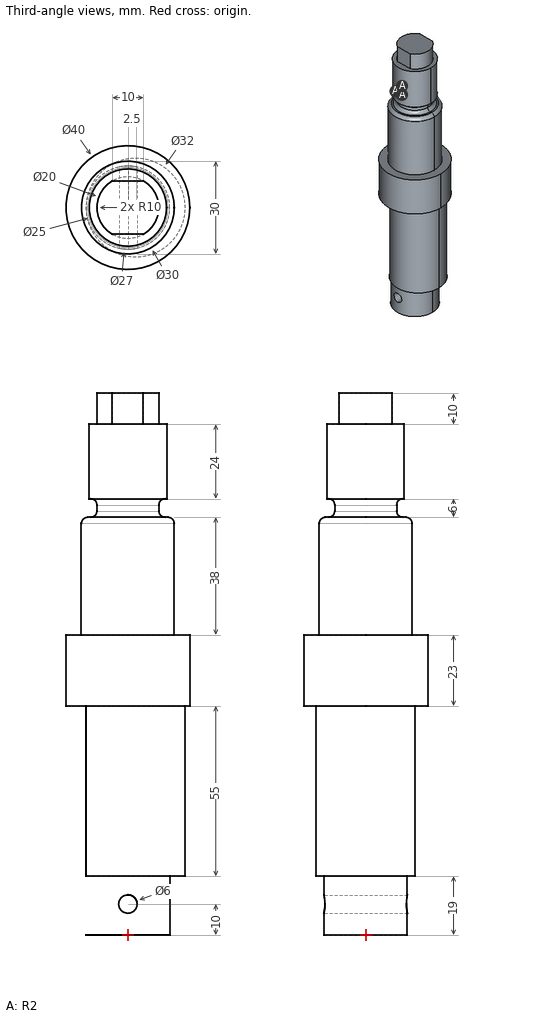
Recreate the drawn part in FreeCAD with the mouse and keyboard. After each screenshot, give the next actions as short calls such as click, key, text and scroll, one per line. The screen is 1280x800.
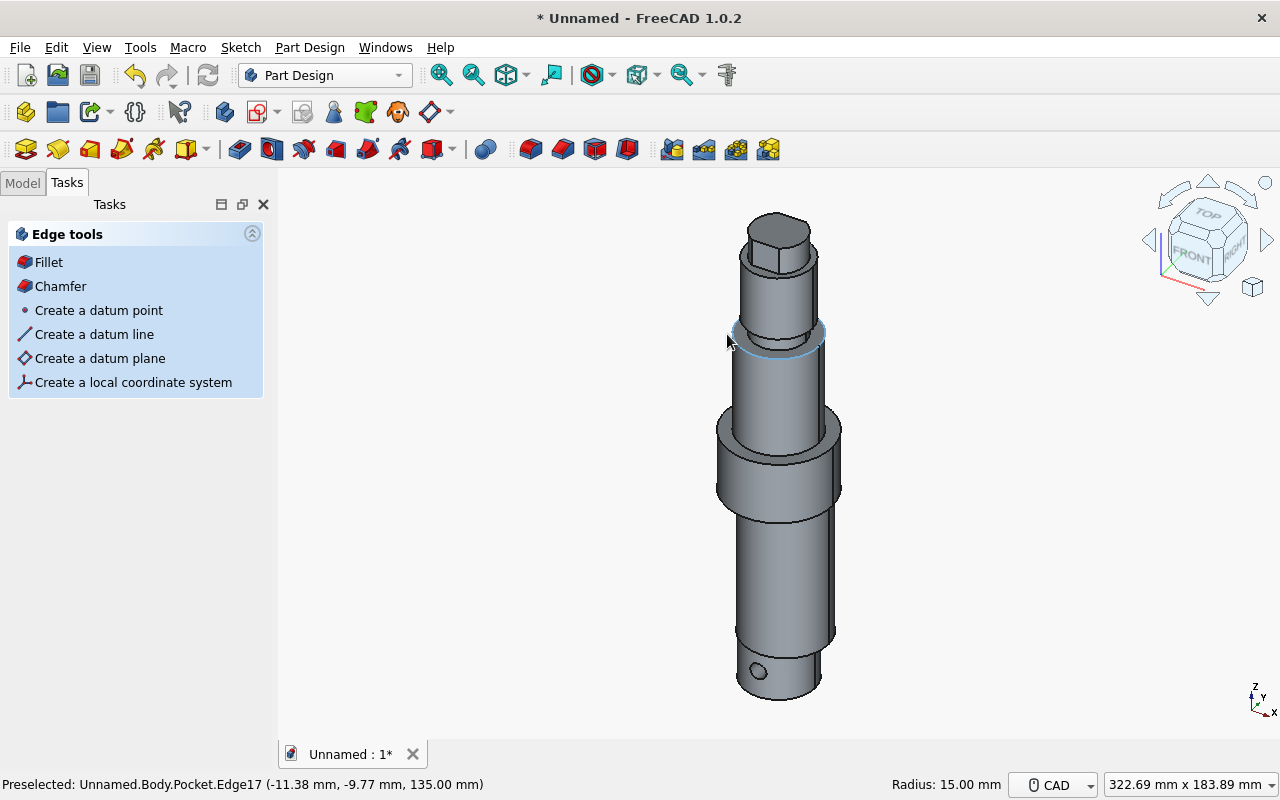
key(0)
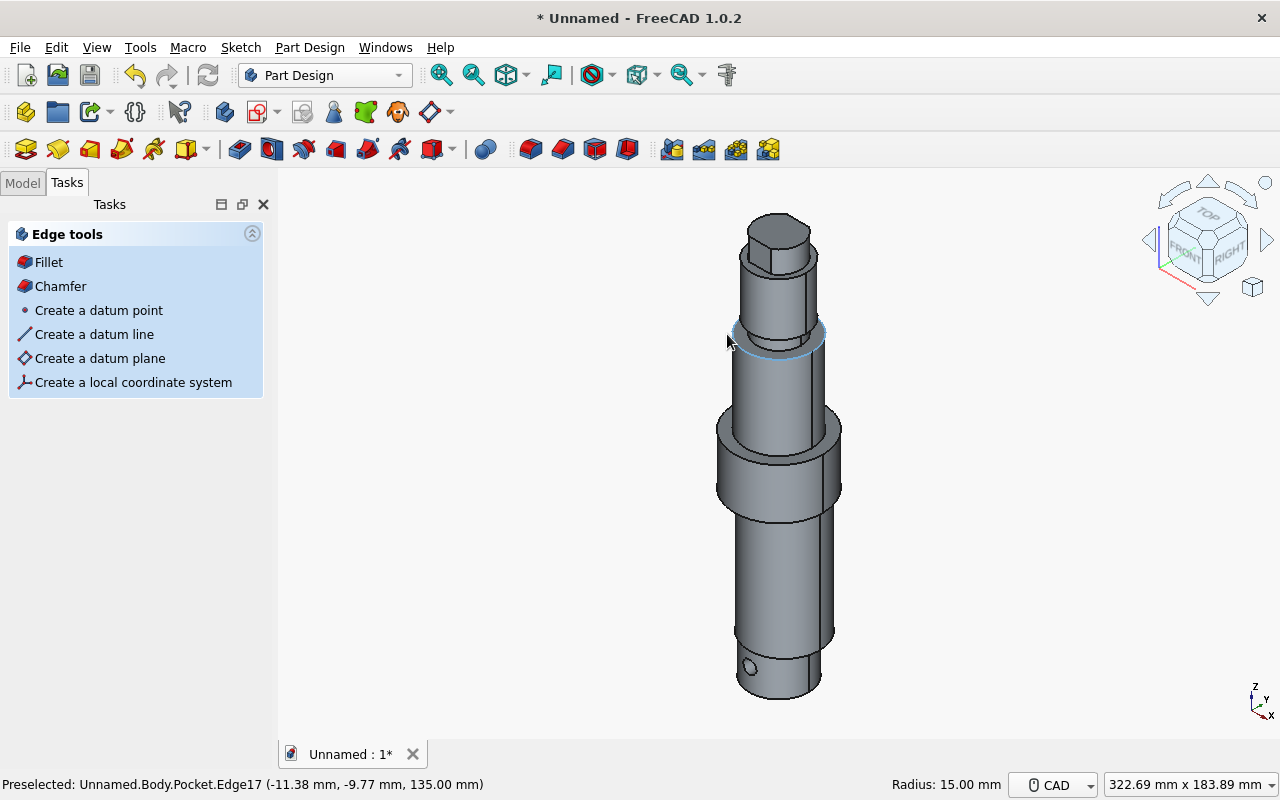
key(2)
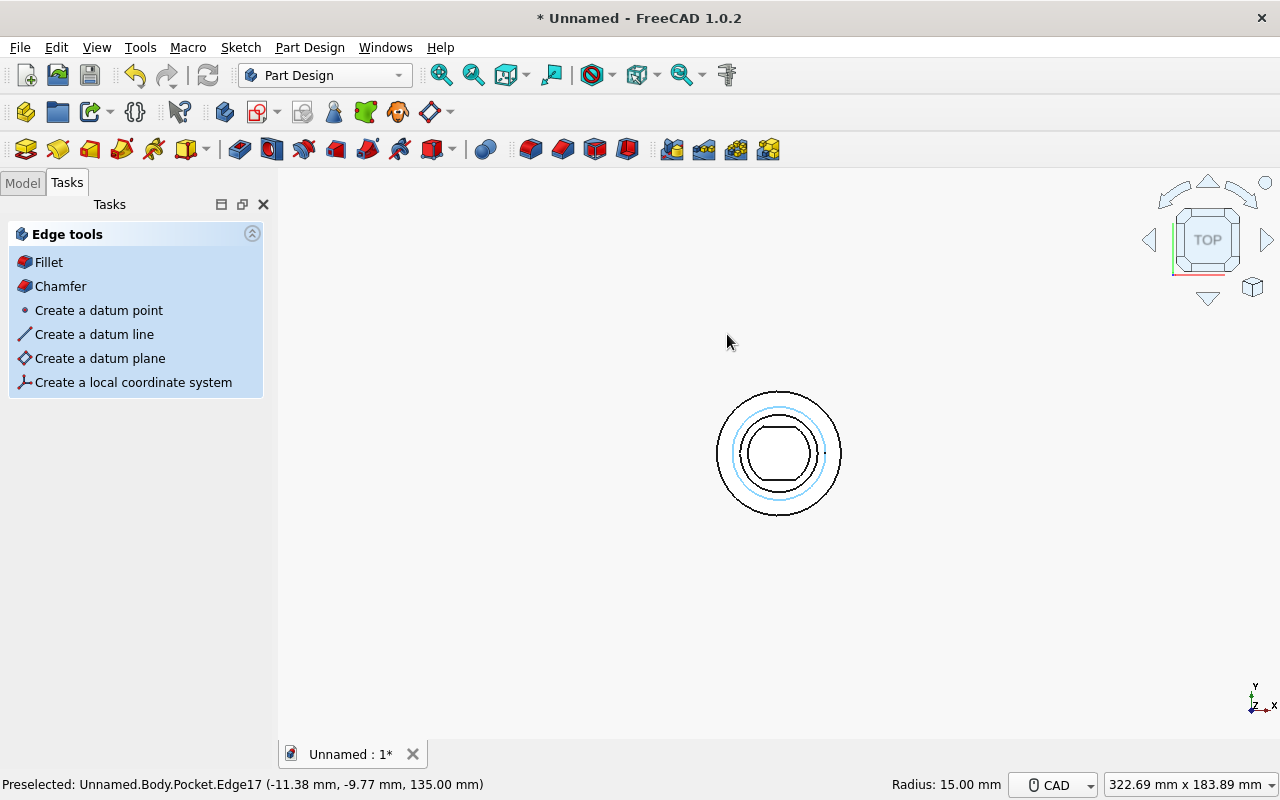
key(v)
key(f)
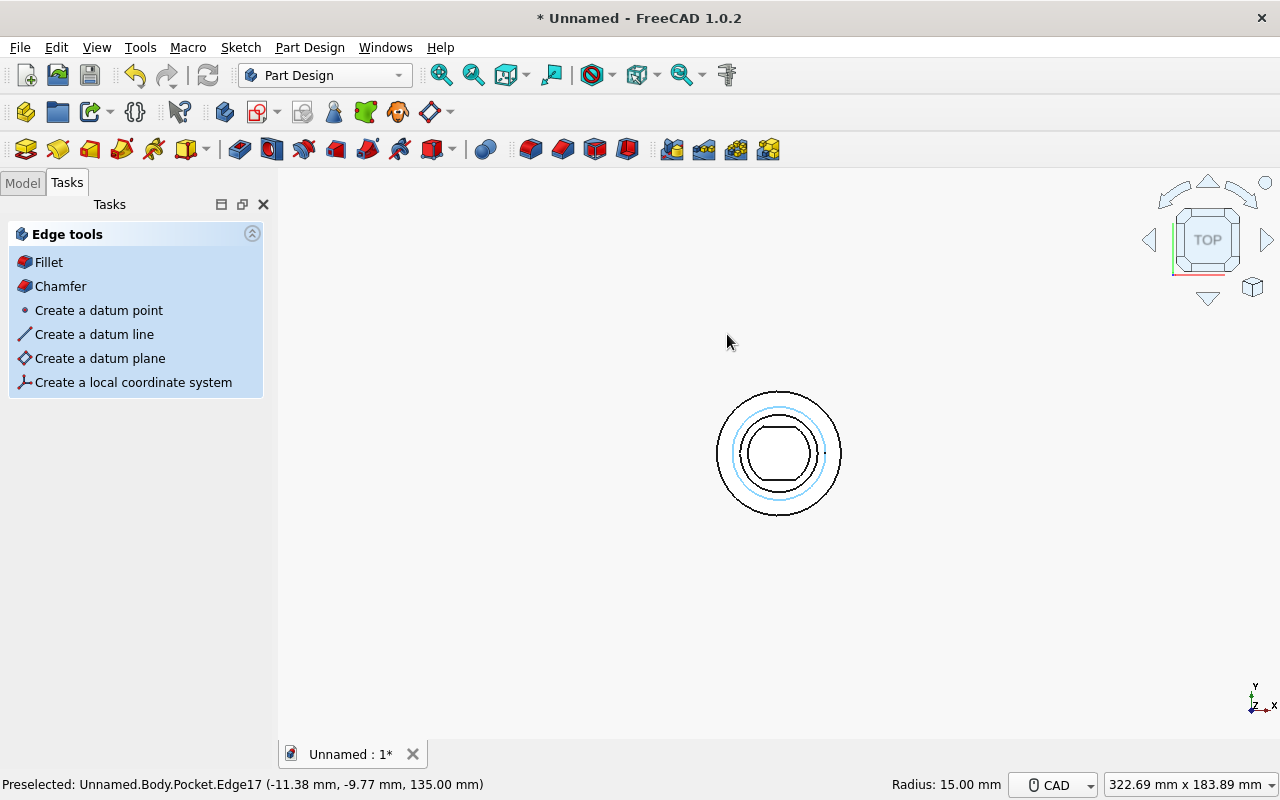
key(1)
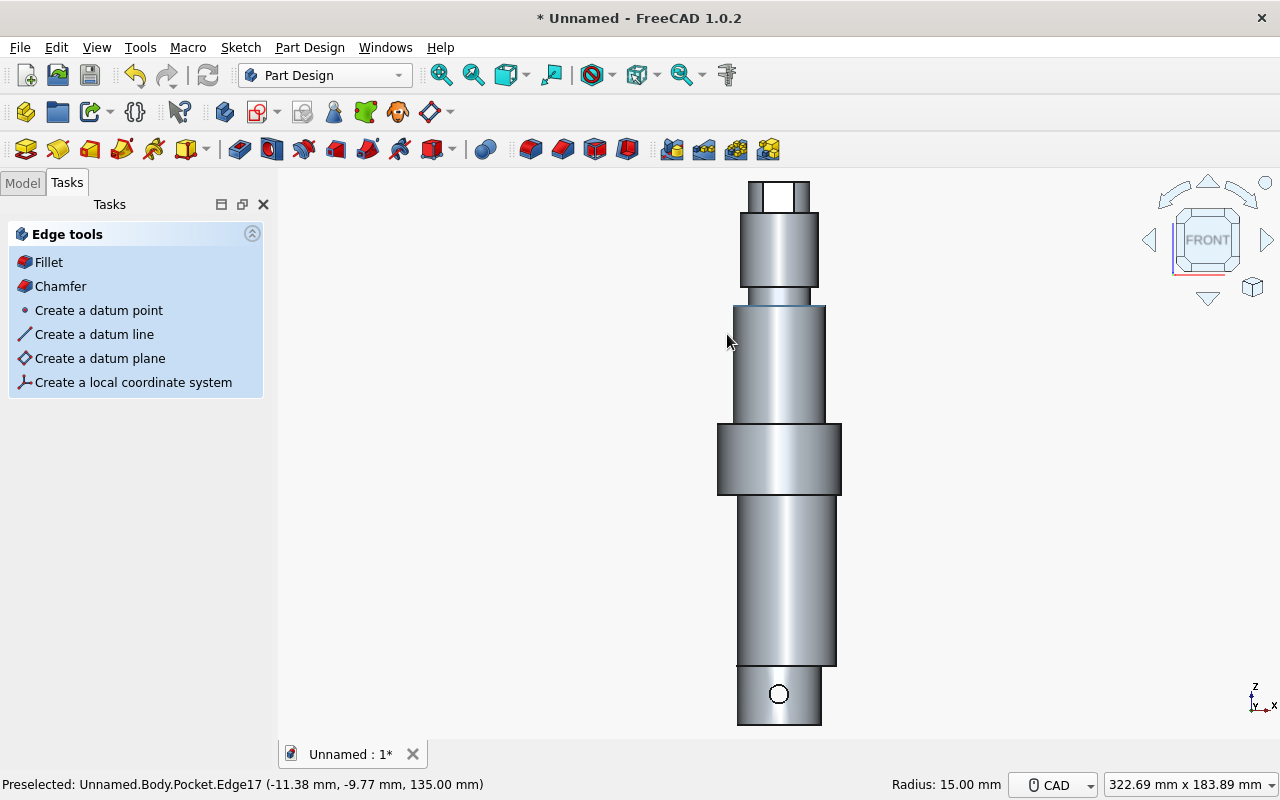
key(3)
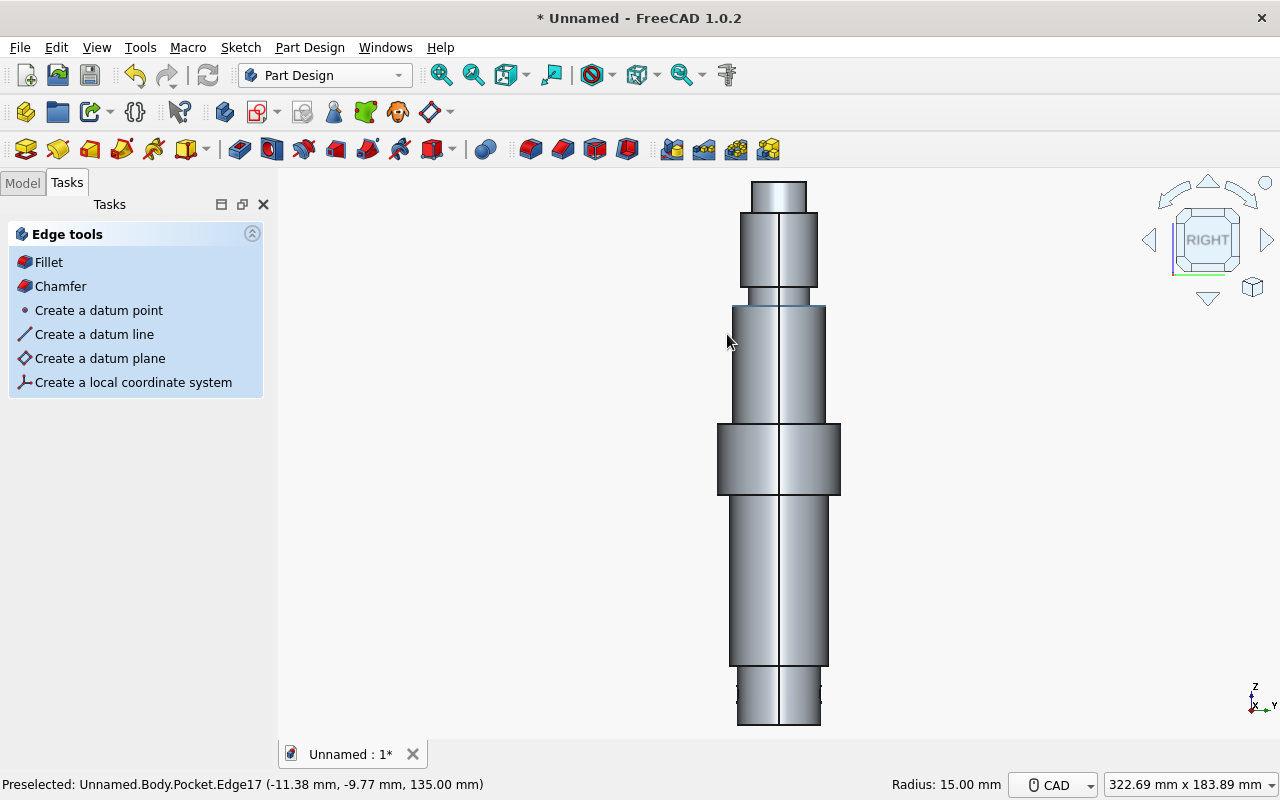
key(5)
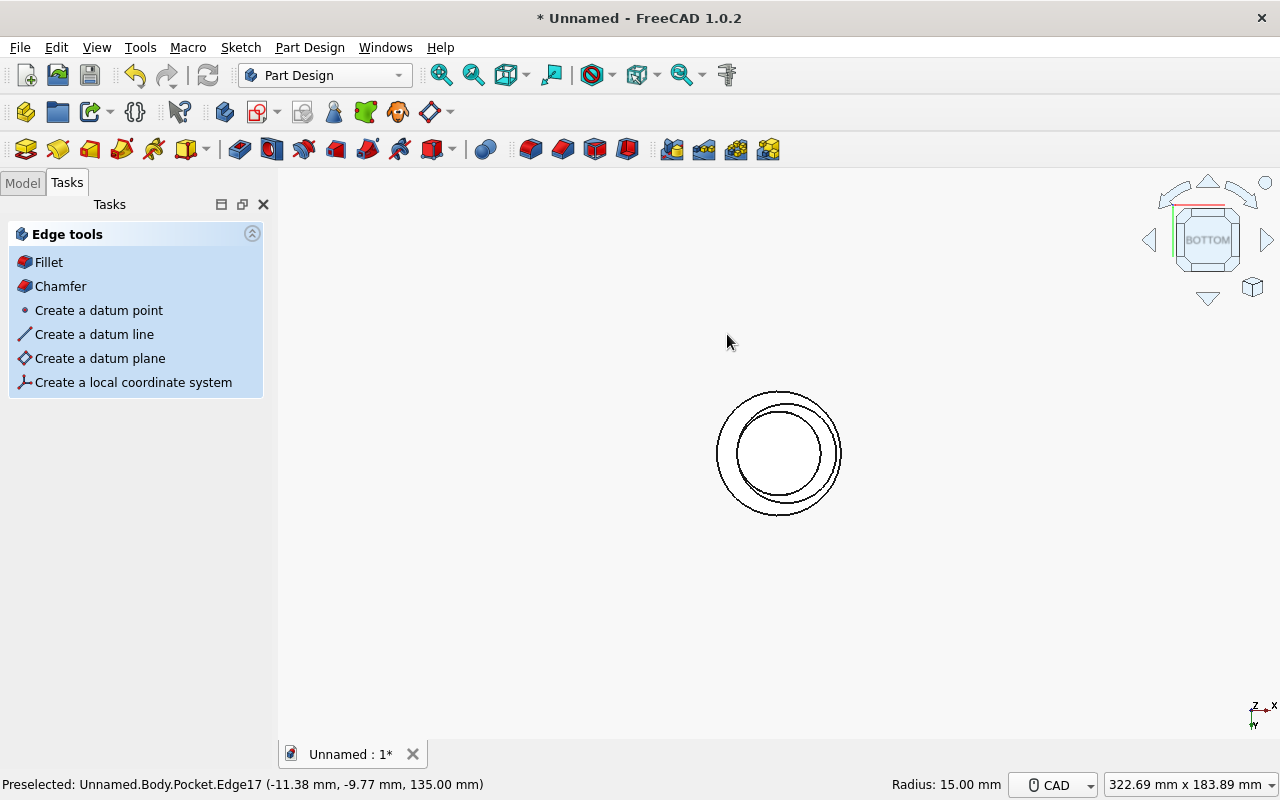
key(v)
key(f)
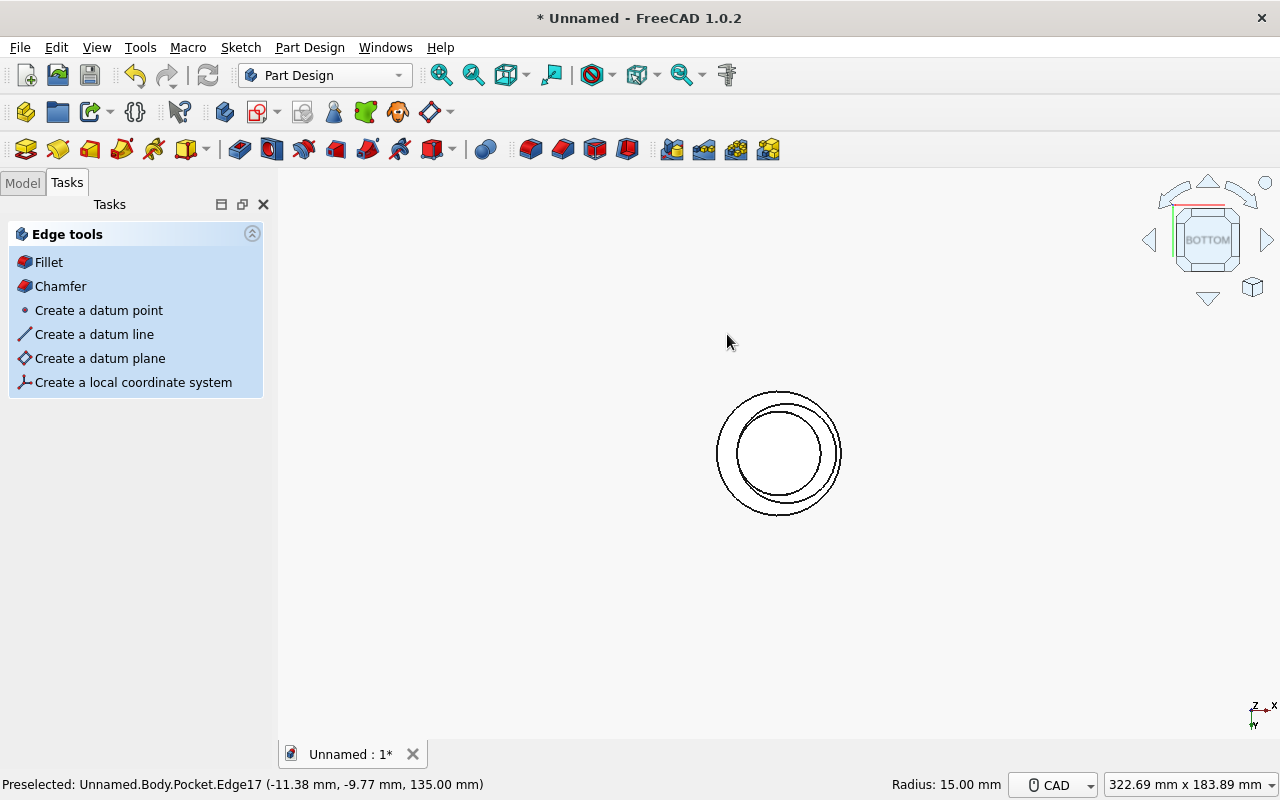
key(4)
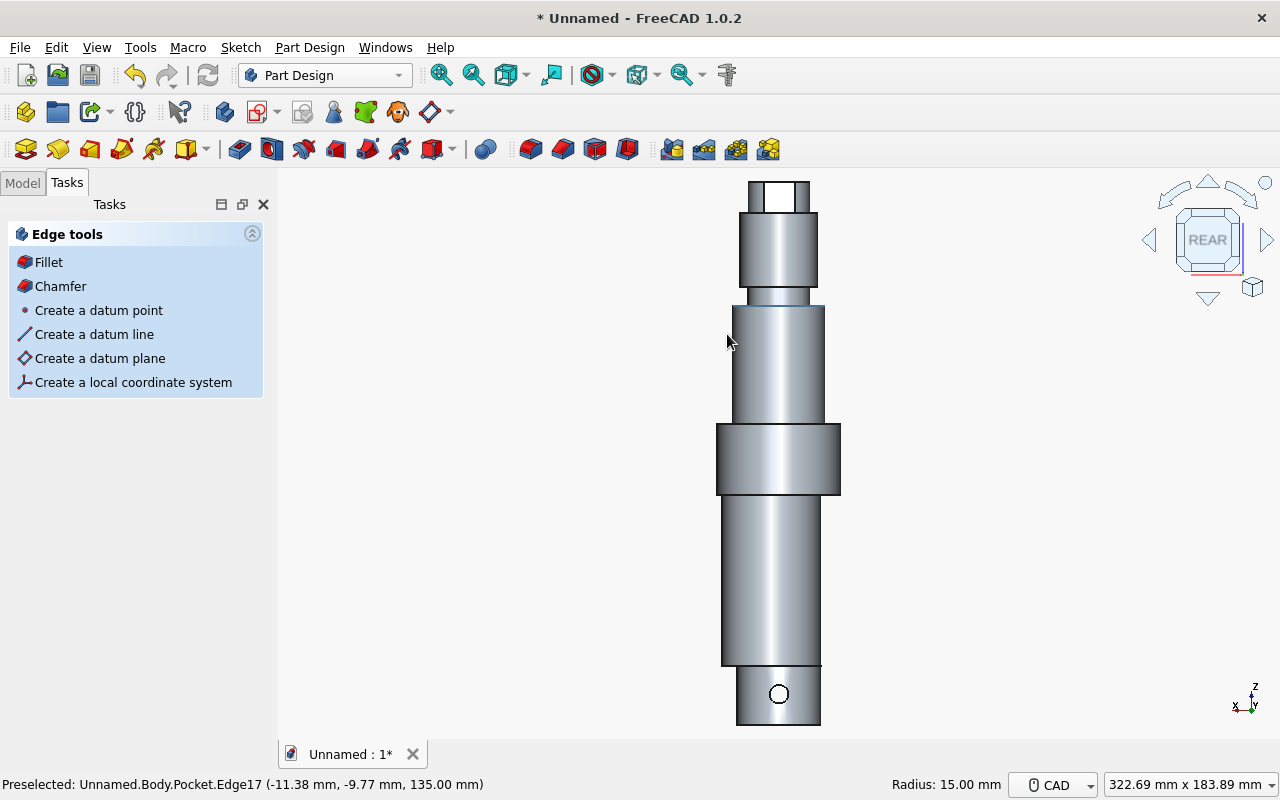
key(6)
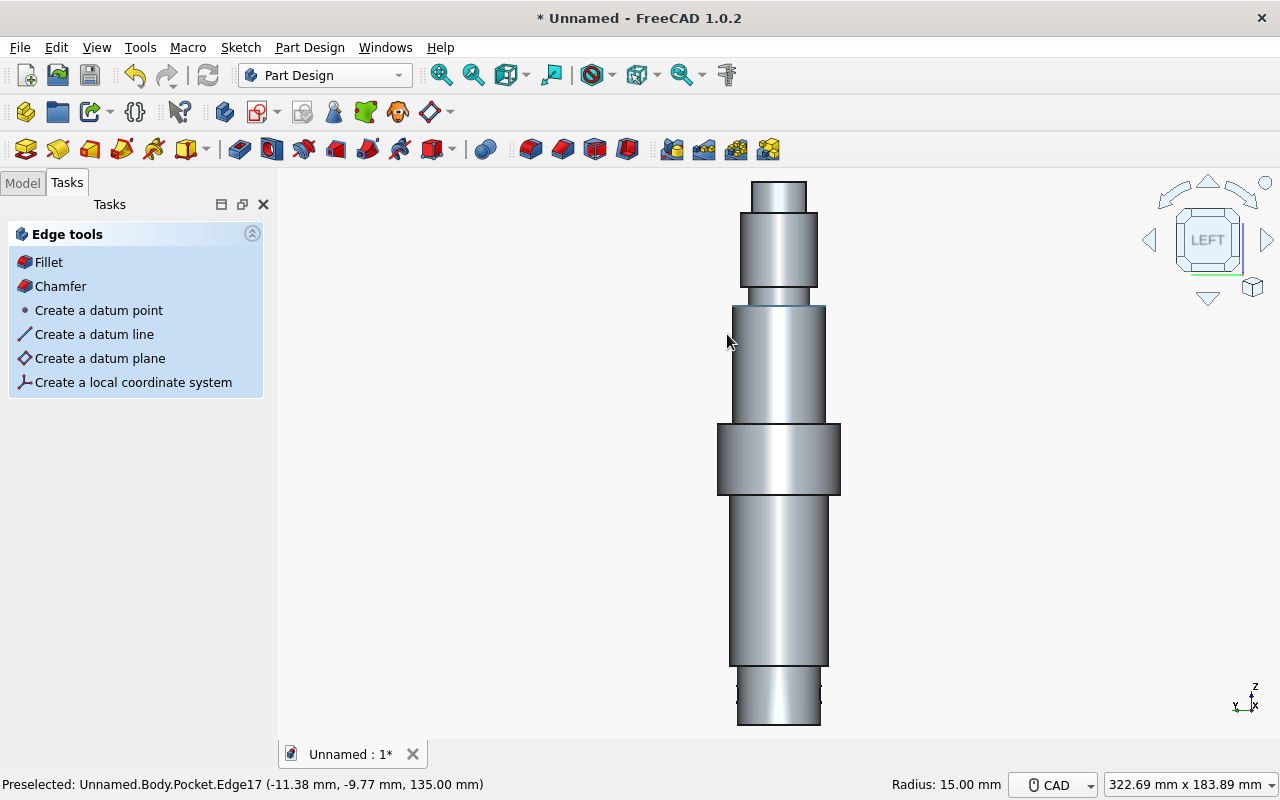
key(v)
key(3)